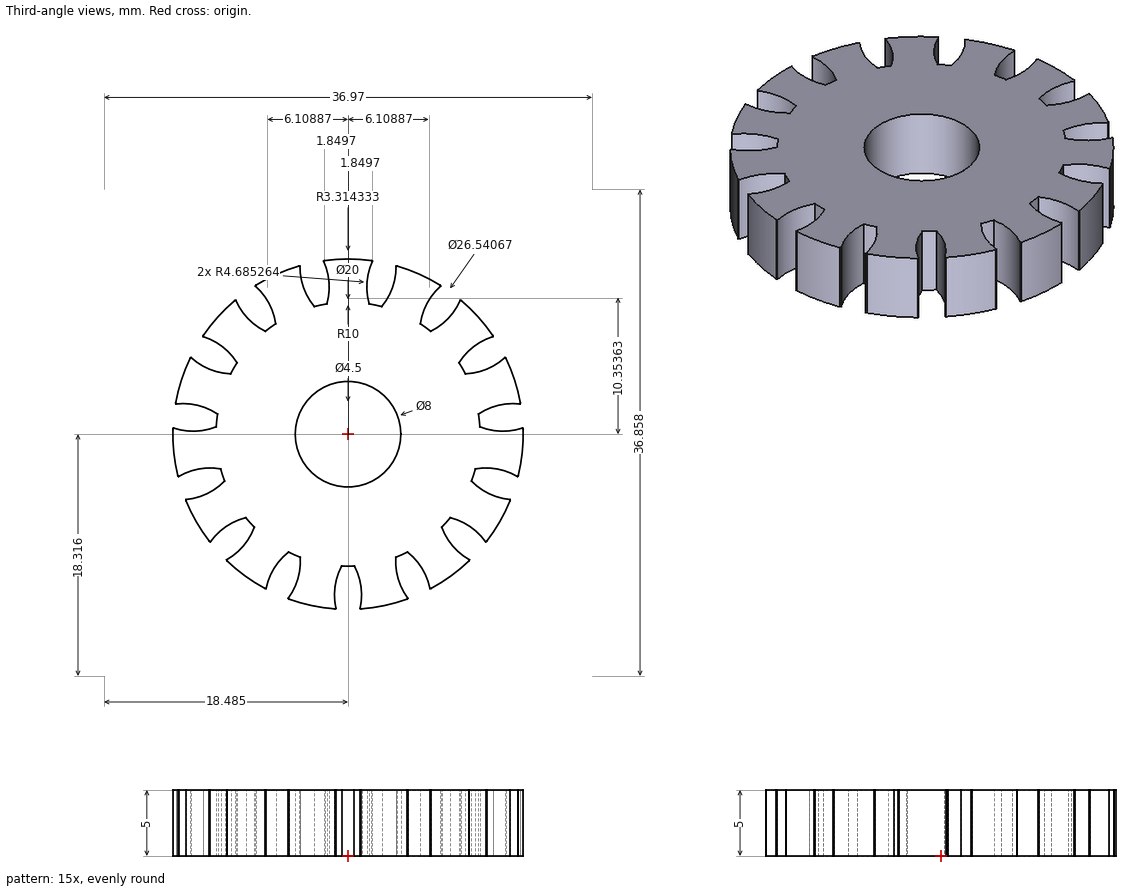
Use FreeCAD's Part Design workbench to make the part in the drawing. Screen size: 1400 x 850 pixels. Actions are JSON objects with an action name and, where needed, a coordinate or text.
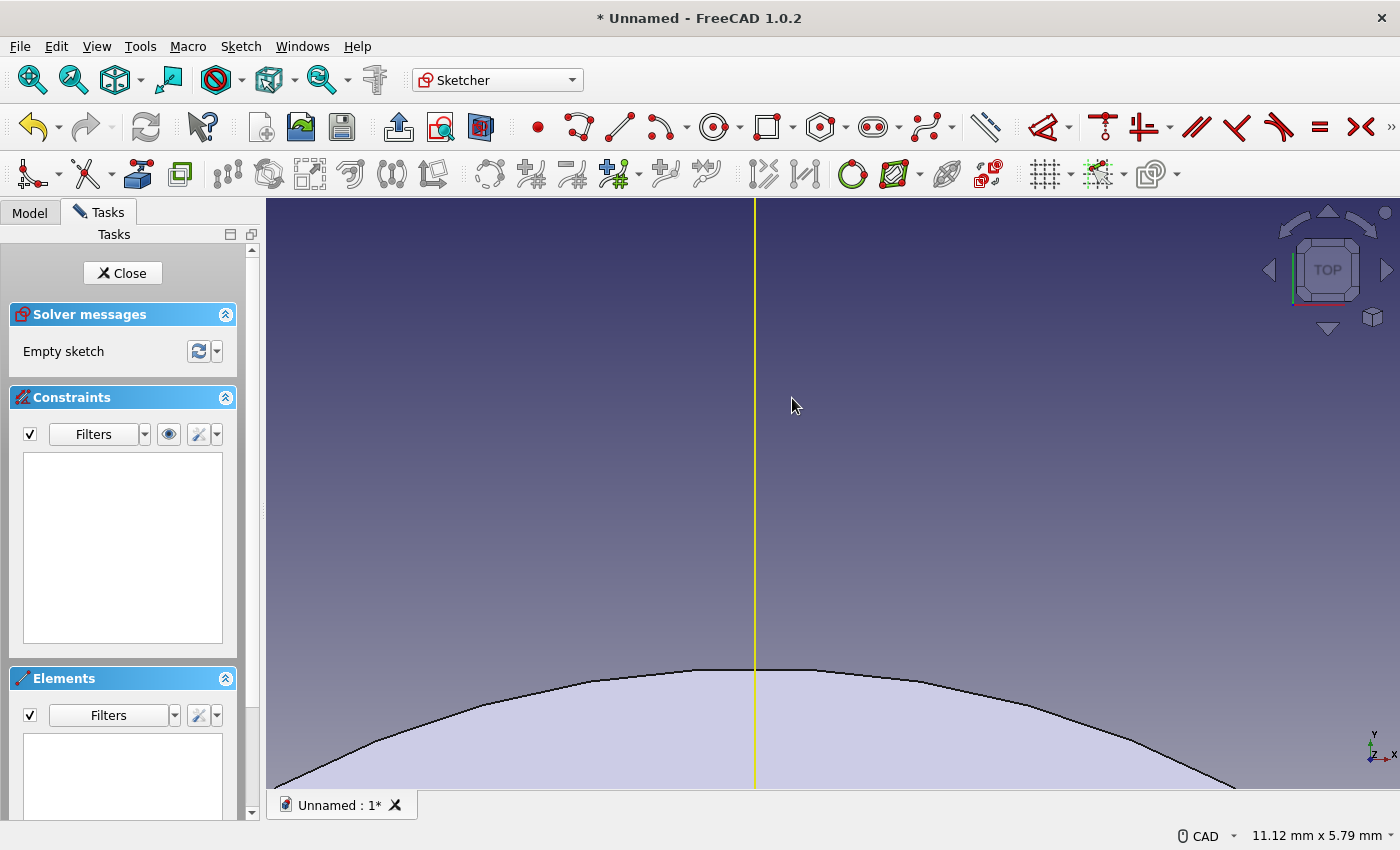
{"action": "key", "text": "g 3 a"}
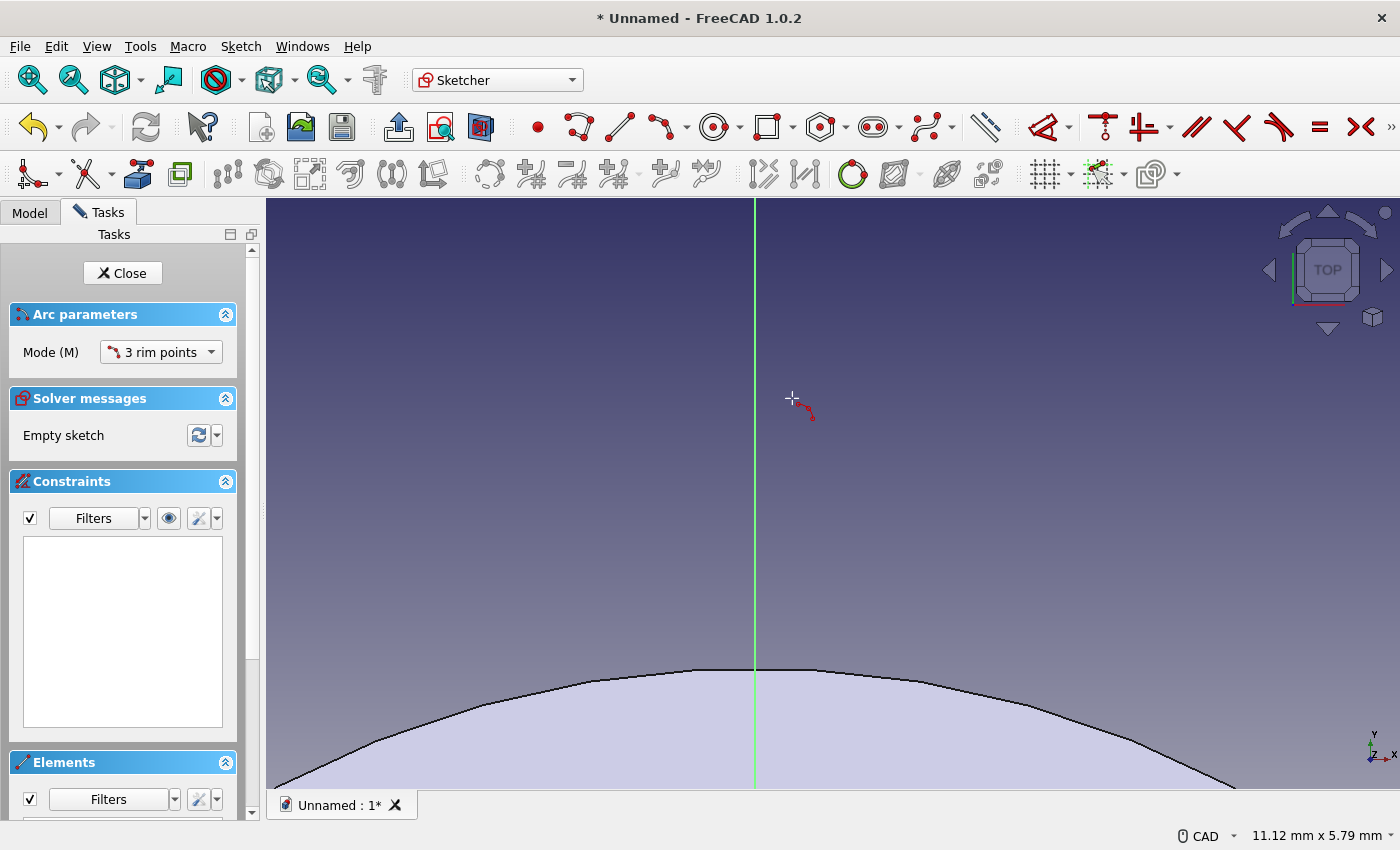
{"action": "left_click", "coordinate": [591, 681]}
{"action": "left_click", "coordinate": [918, 681]}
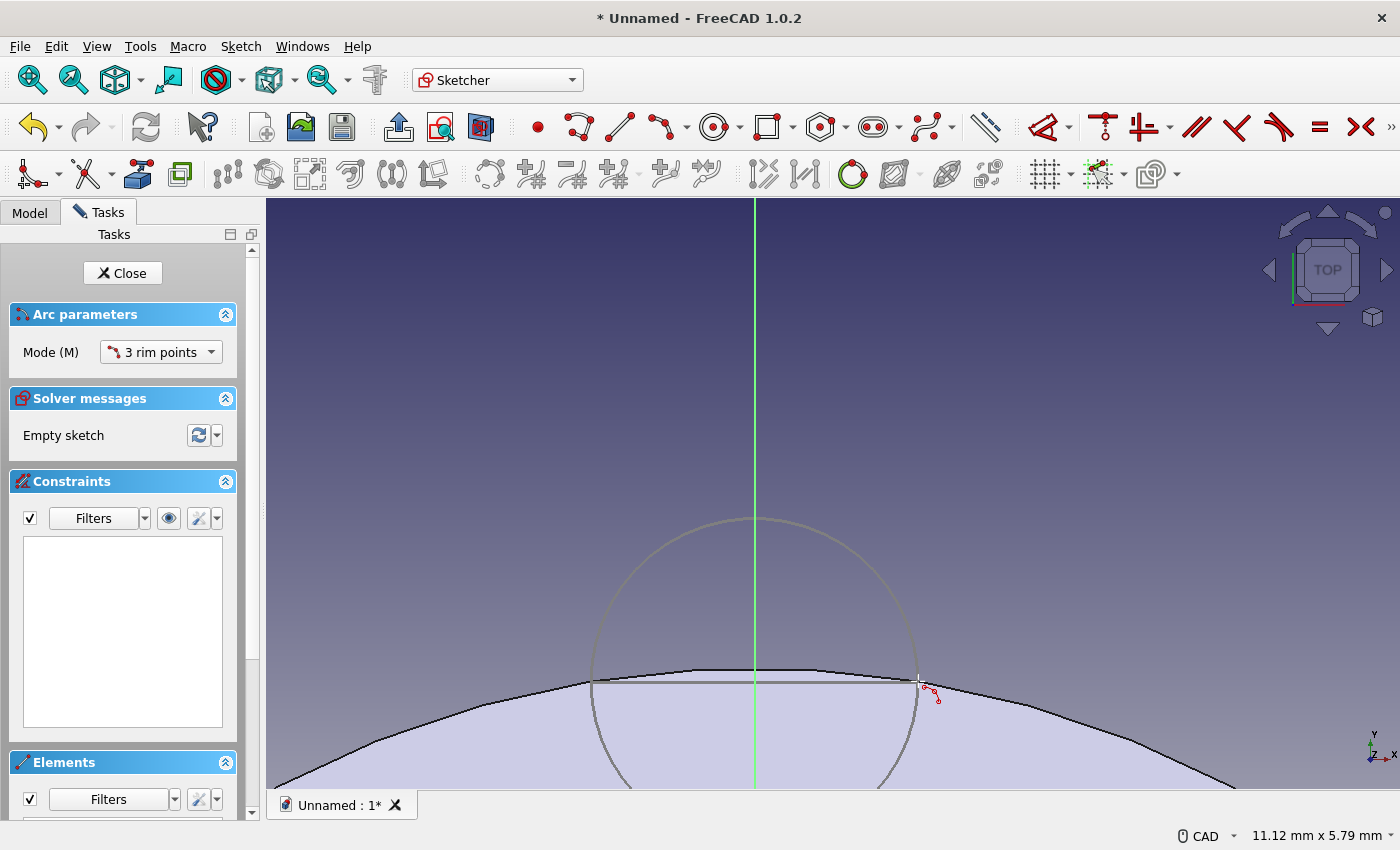
{"action": "scroll", "coordinate": [788, 669], "scroll_direction": "up", "scroll_amount": 2}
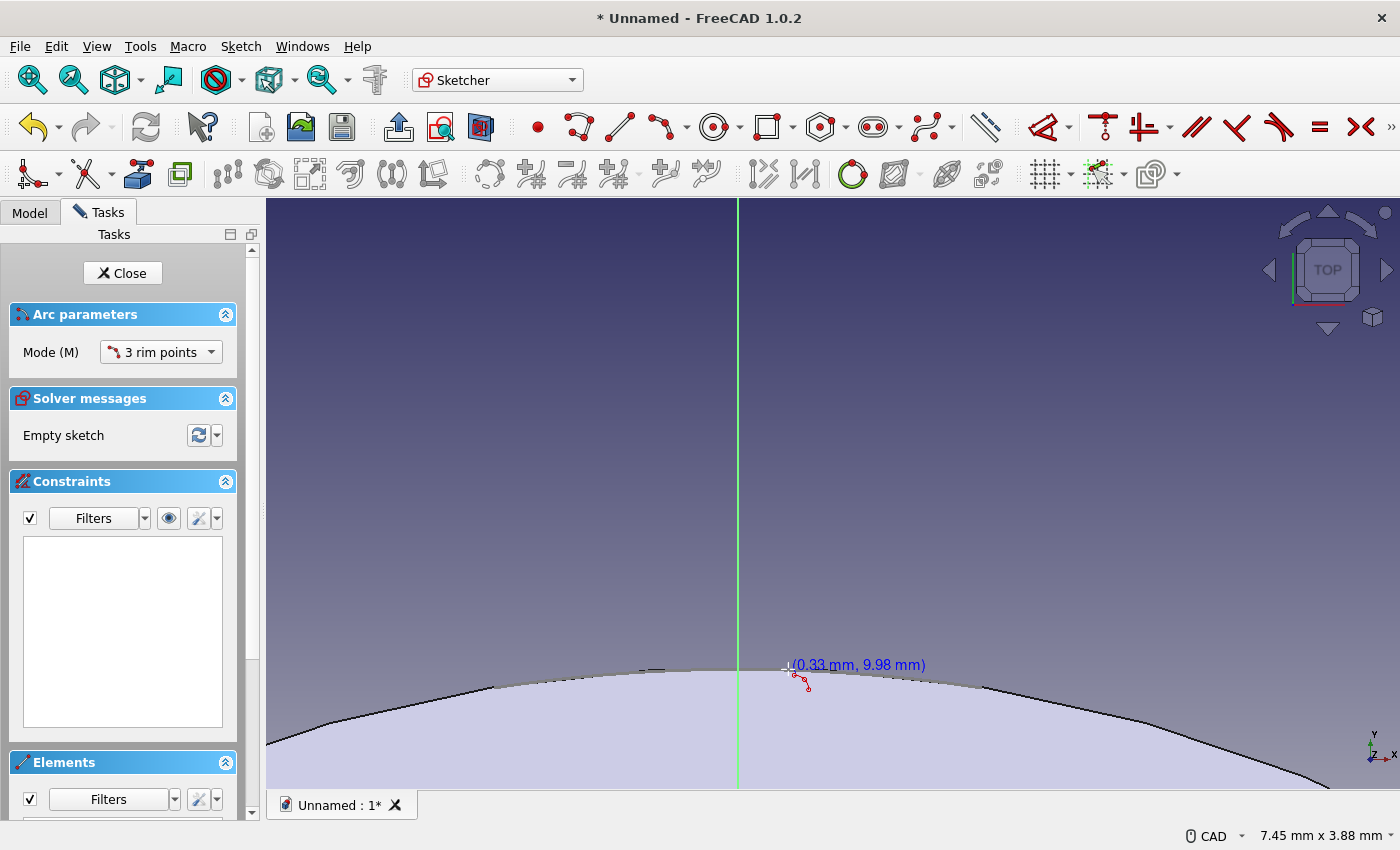
{"action": "left_click", "coordinate": [787, 668]}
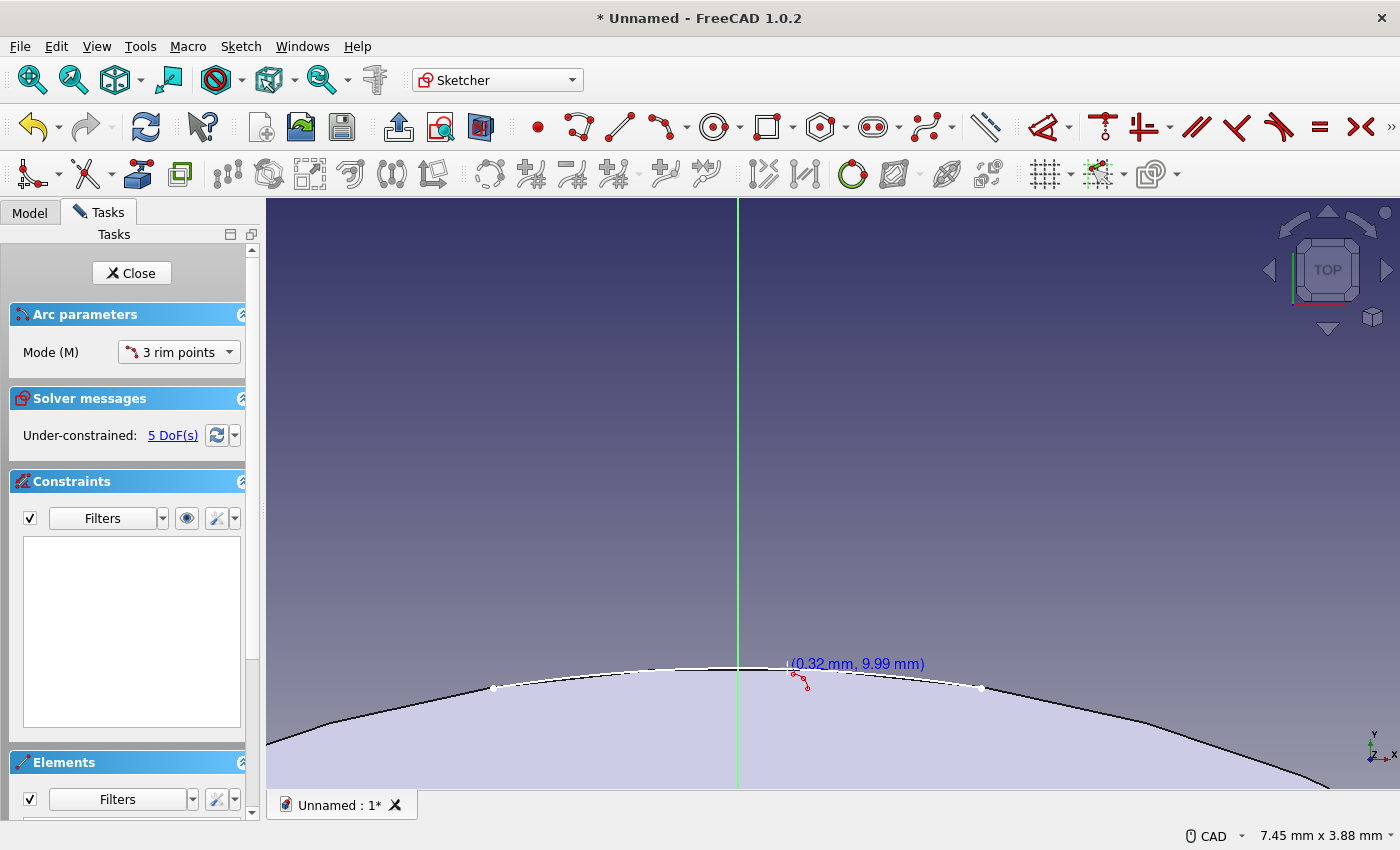
{"action": "left_click", "coordinate": [982, 688]}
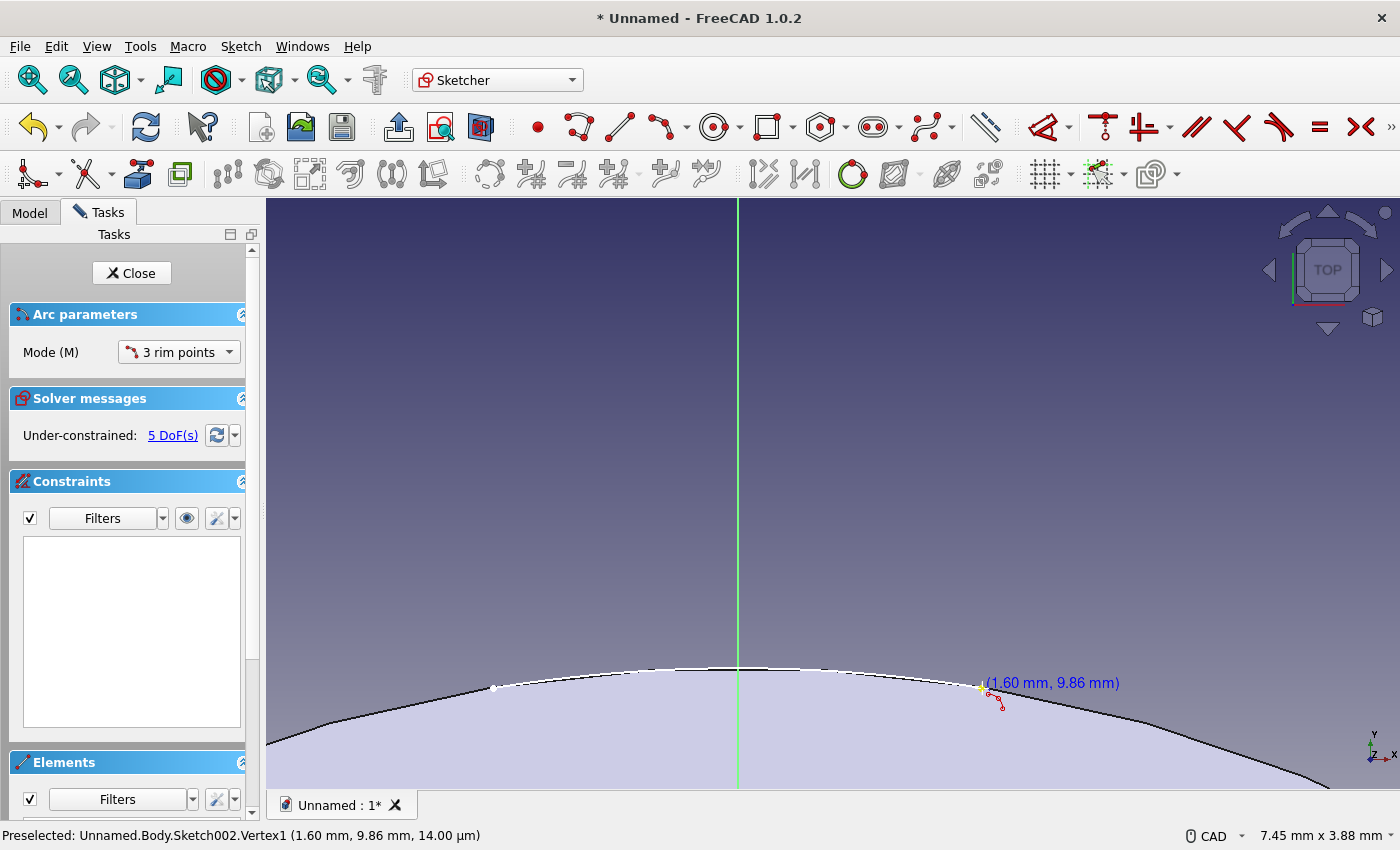
{"action": "scroll", "coordinate": [818, 687], "scroll_direction": "down", "scroll_amount": 2}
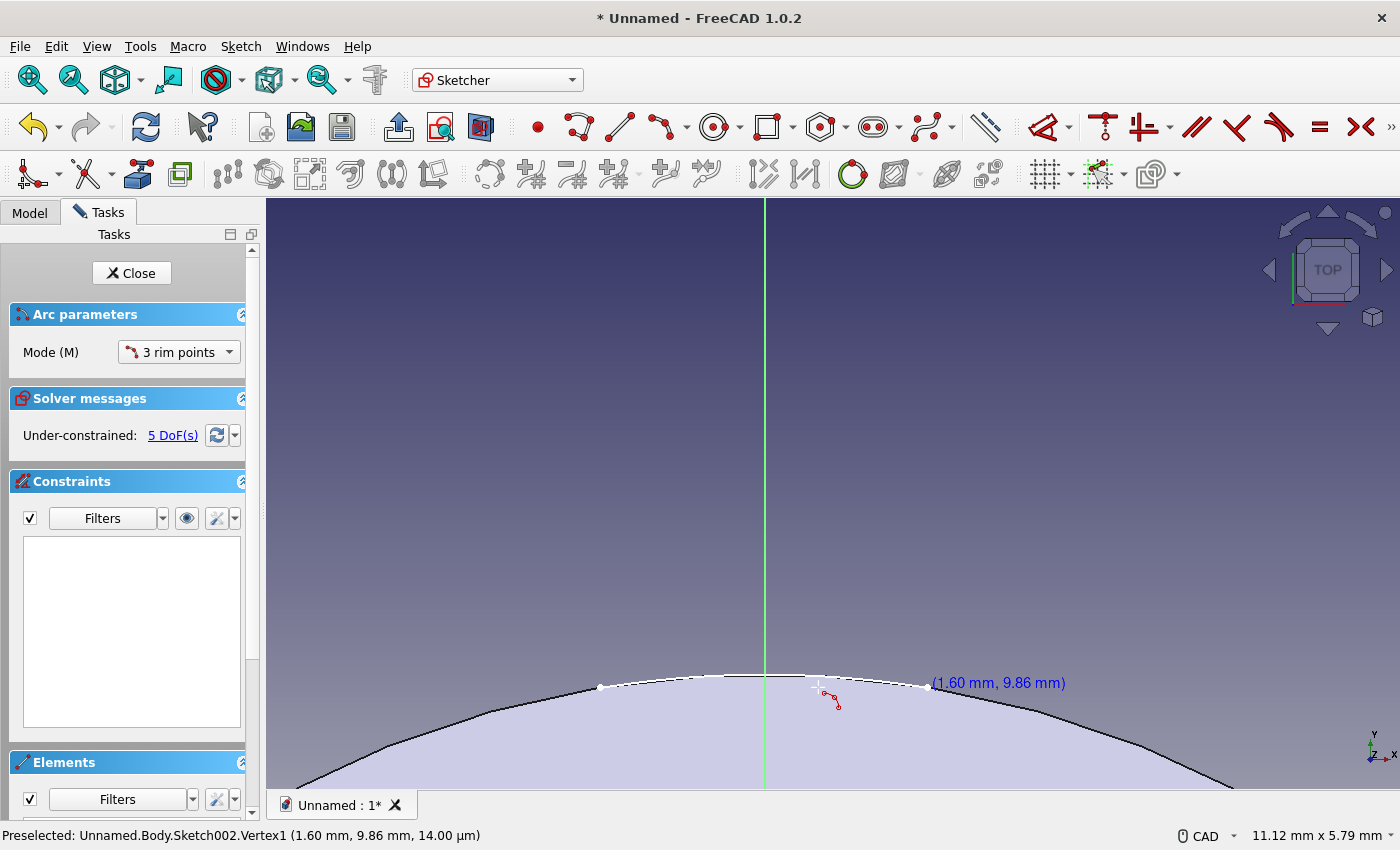
{"action": "left_click", "coordinate": [953, 358]}
{"action": "left_click", "coordinate": [911, 520]}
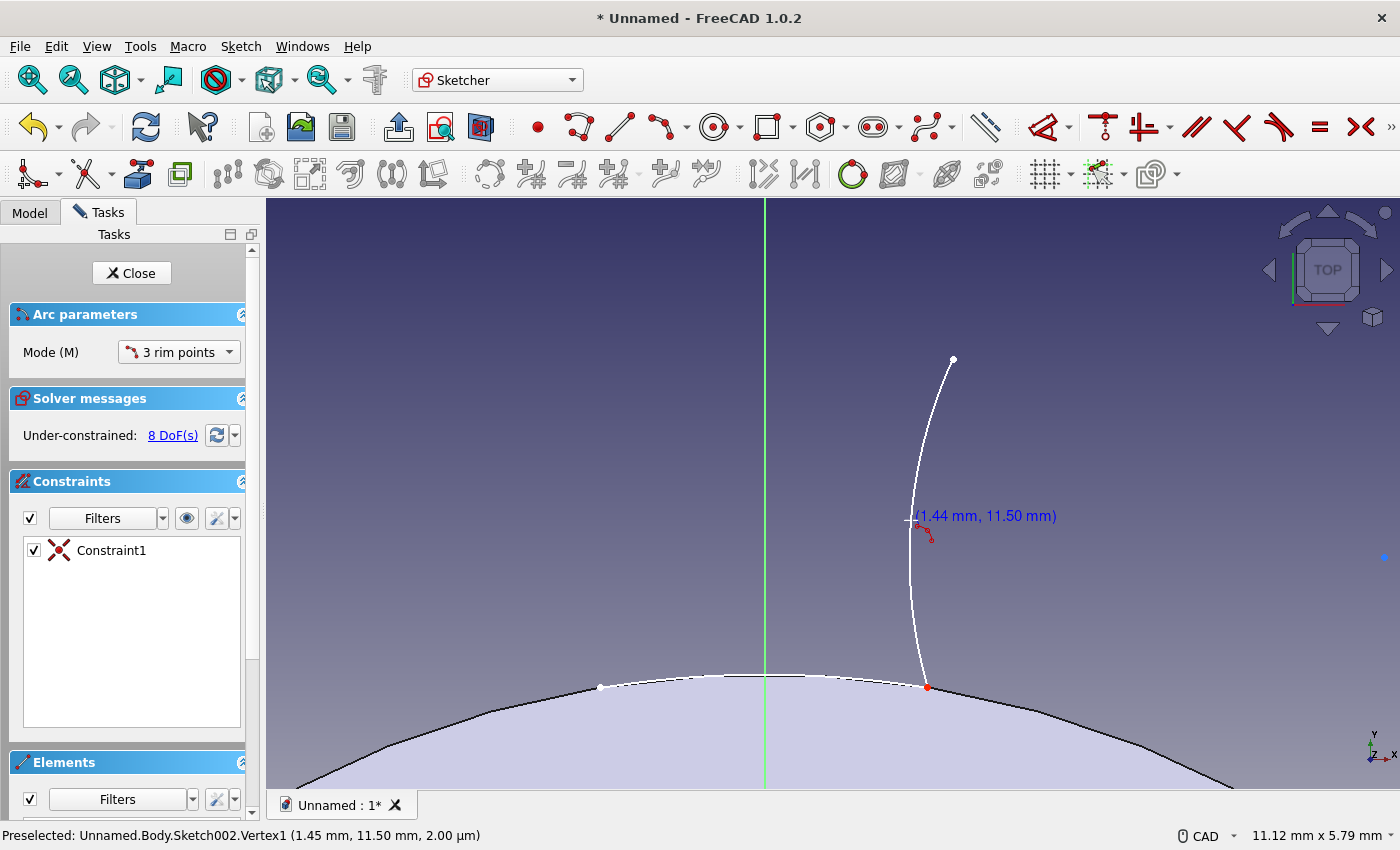
{"action": "left_click", "coordinate": [953, 359]}
{"action": "left_click", "coordinate": [576, 358]}
{"action": "left_click", "coordinate": [805, 302]}